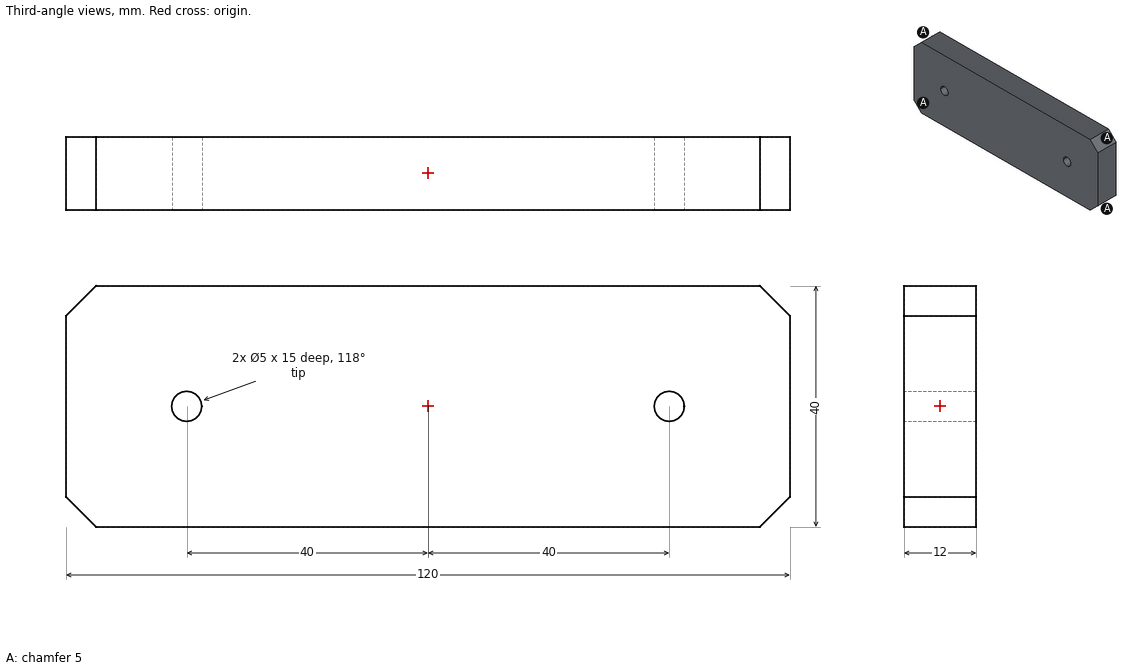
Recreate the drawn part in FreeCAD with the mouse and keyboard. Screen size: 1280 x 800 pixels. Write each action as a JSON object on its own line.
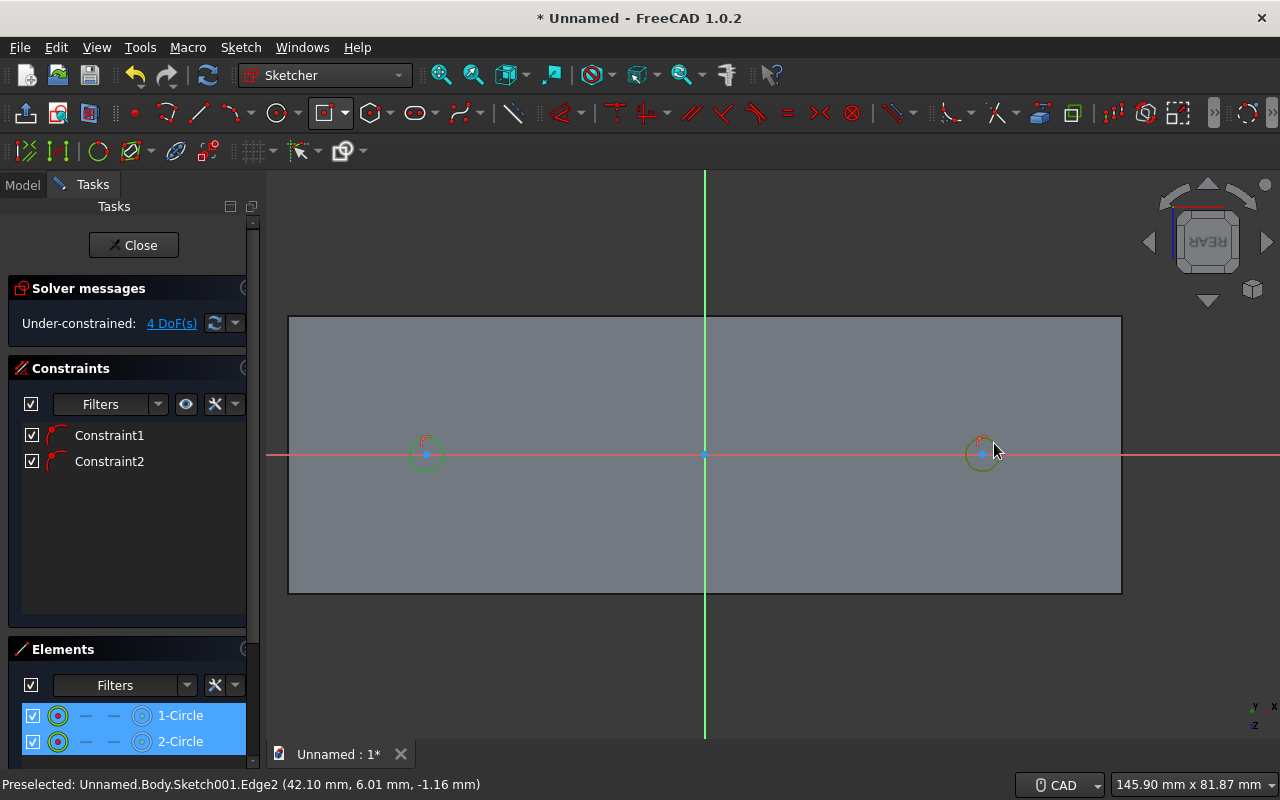
{"action": "left_click", "coordinate": [788, 114]}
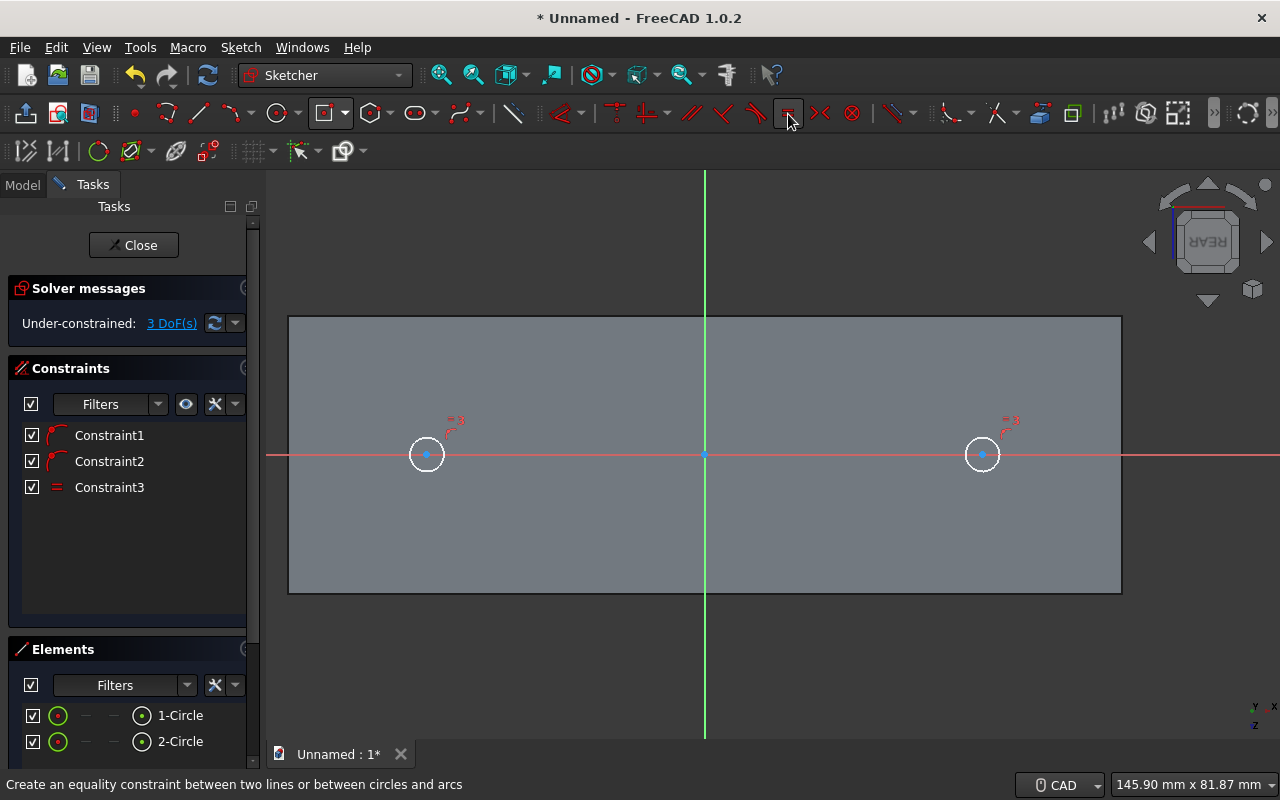
{"action": "left_click", "coordinate": [560, 114]}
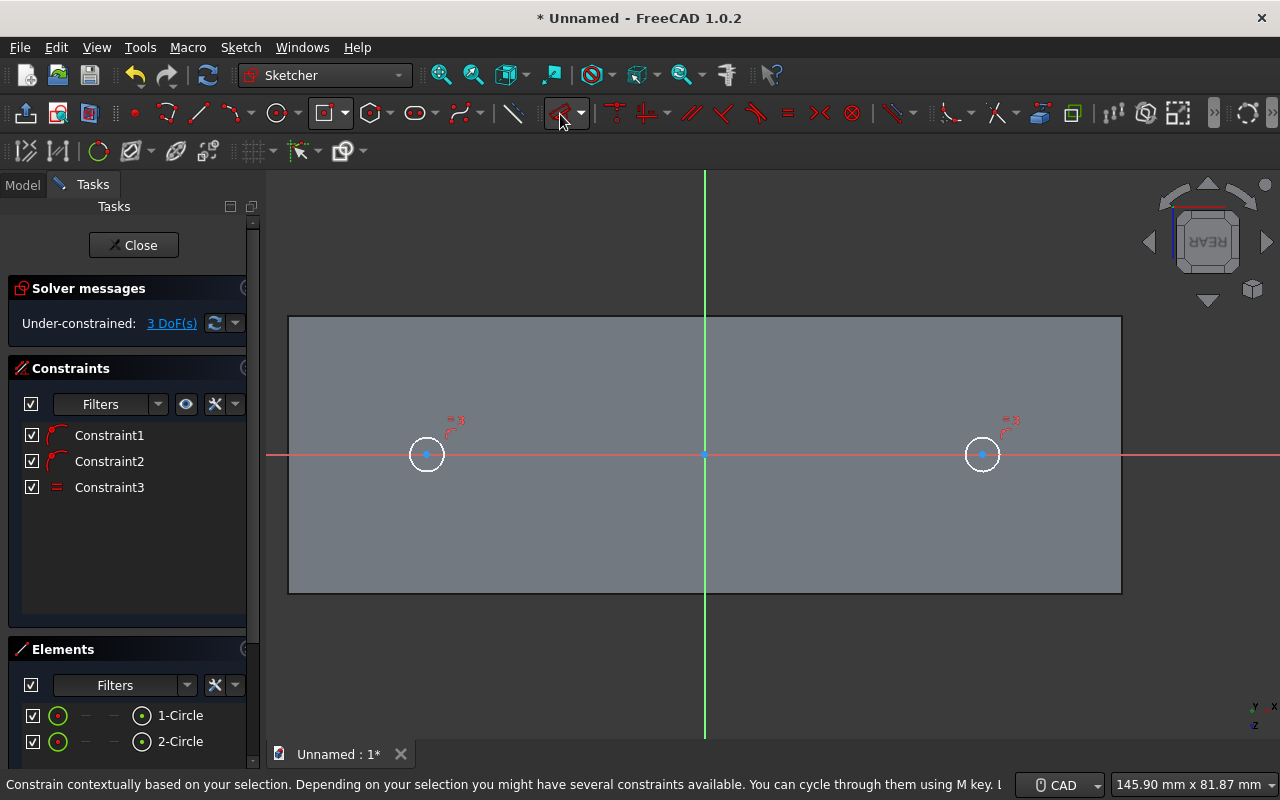
{"action": "left_click", "coordinate": [439, 443]}
{"action": "left_click", "coordinate": [462, 421]}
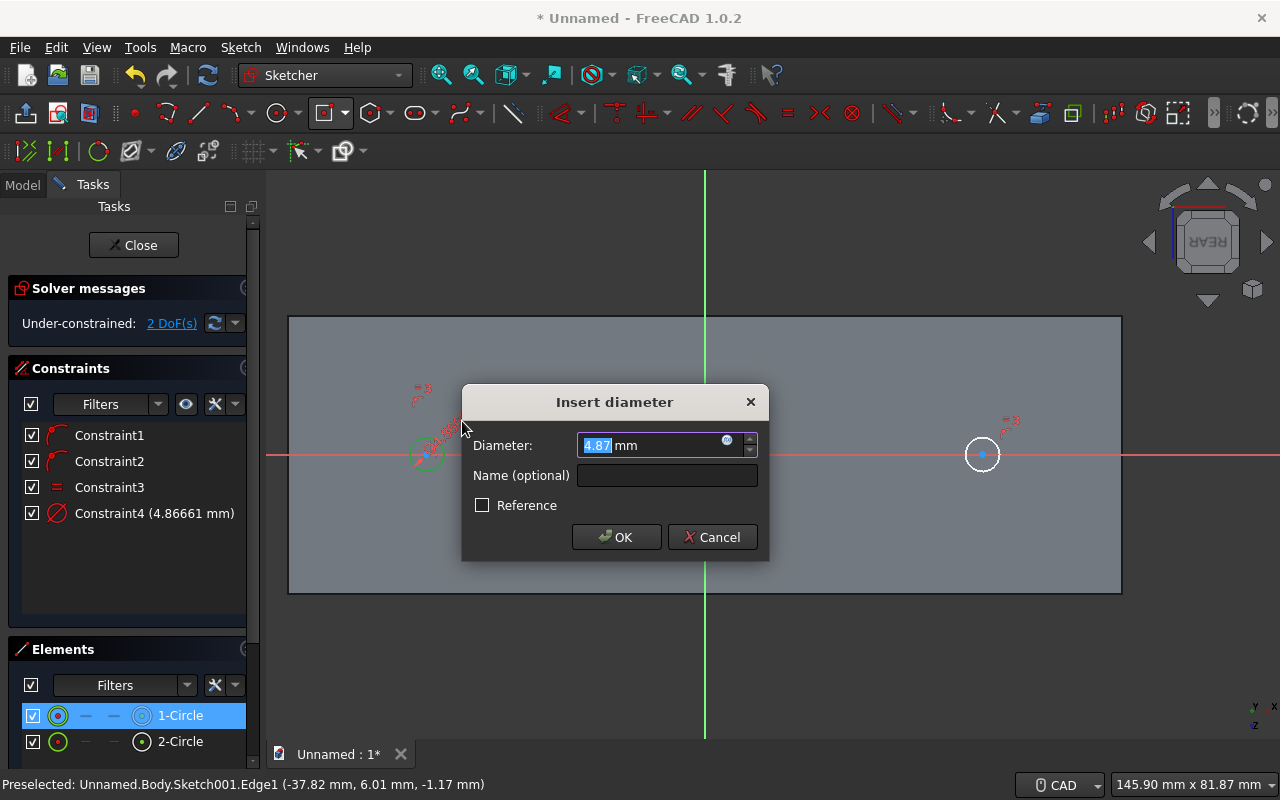
{"action": "type", "text": "5"}
{"action": "key", "text": "Return"}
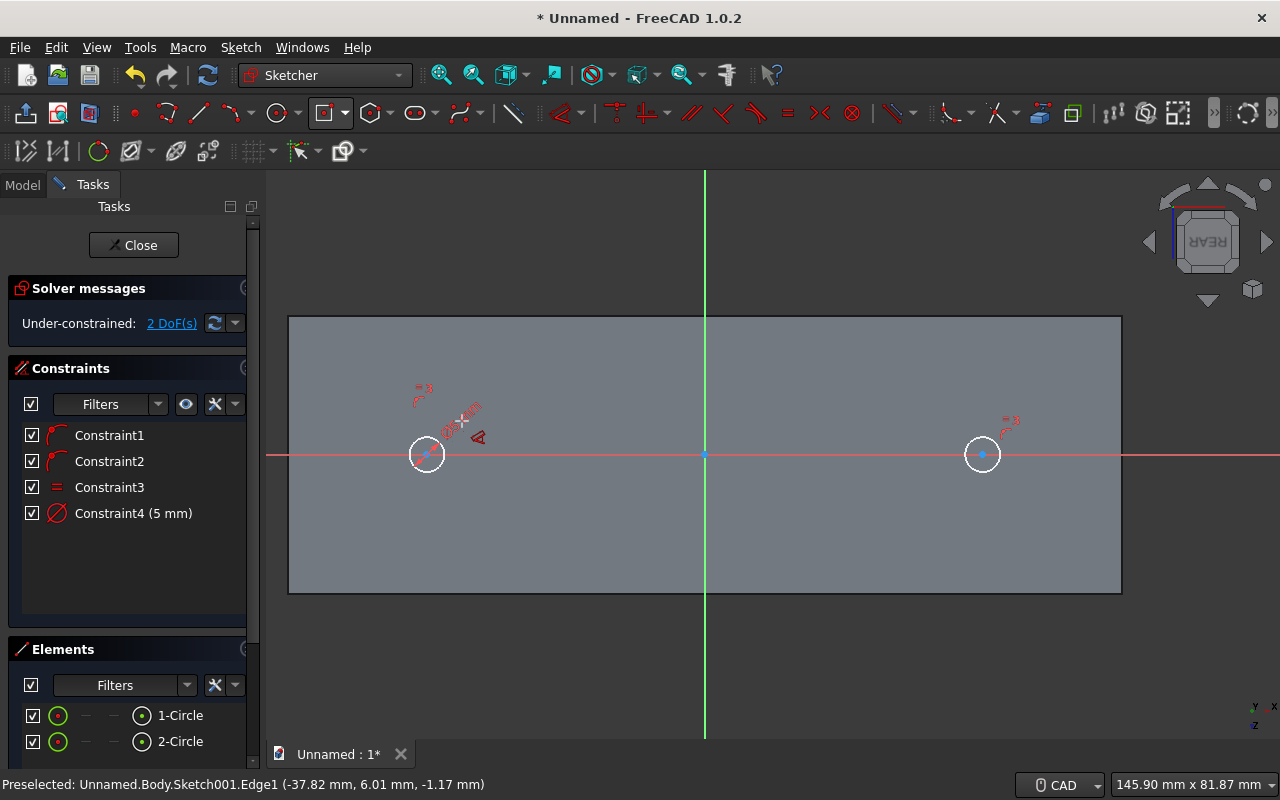
{"action": "left_click", "coordinate": [427, 455]}
{"action": "left_click", "coordinate": [566, 489]}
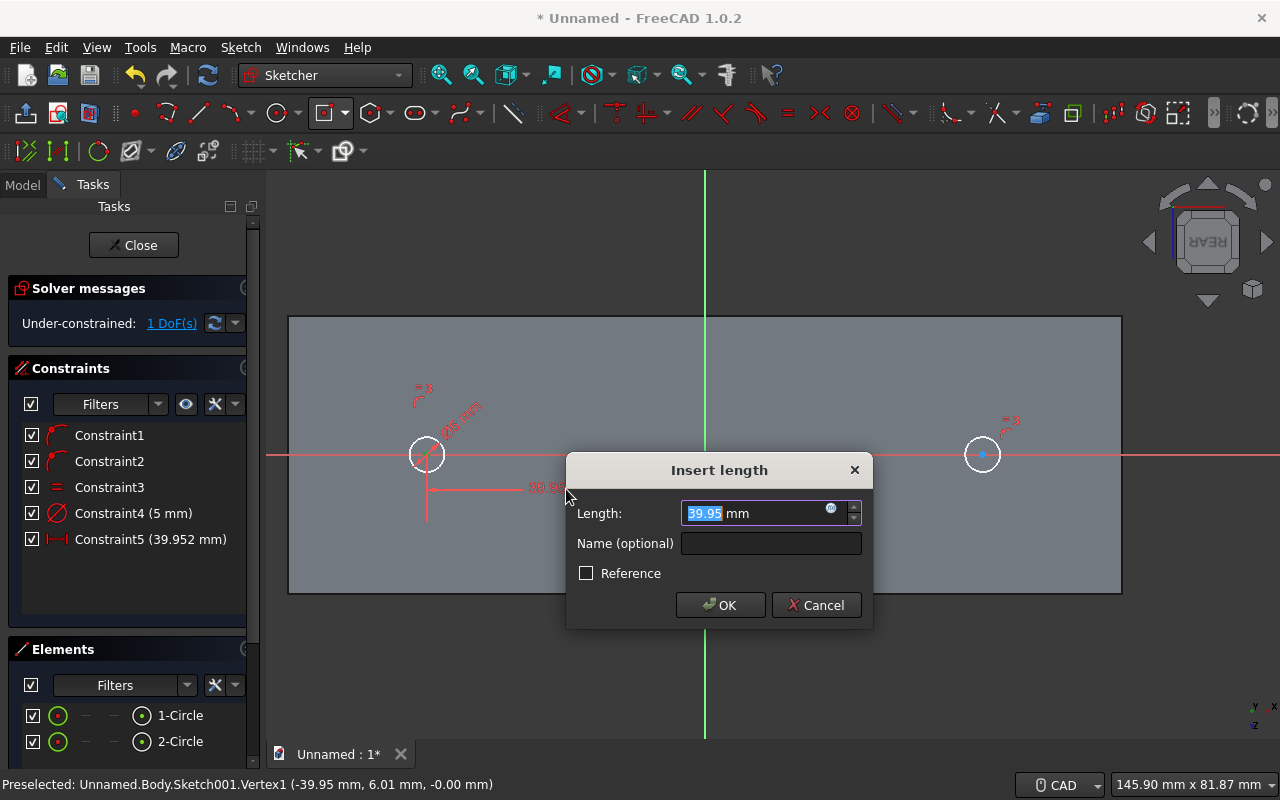
{"action": "type", "text": "40"}
{"action": "key", "text": "Return"}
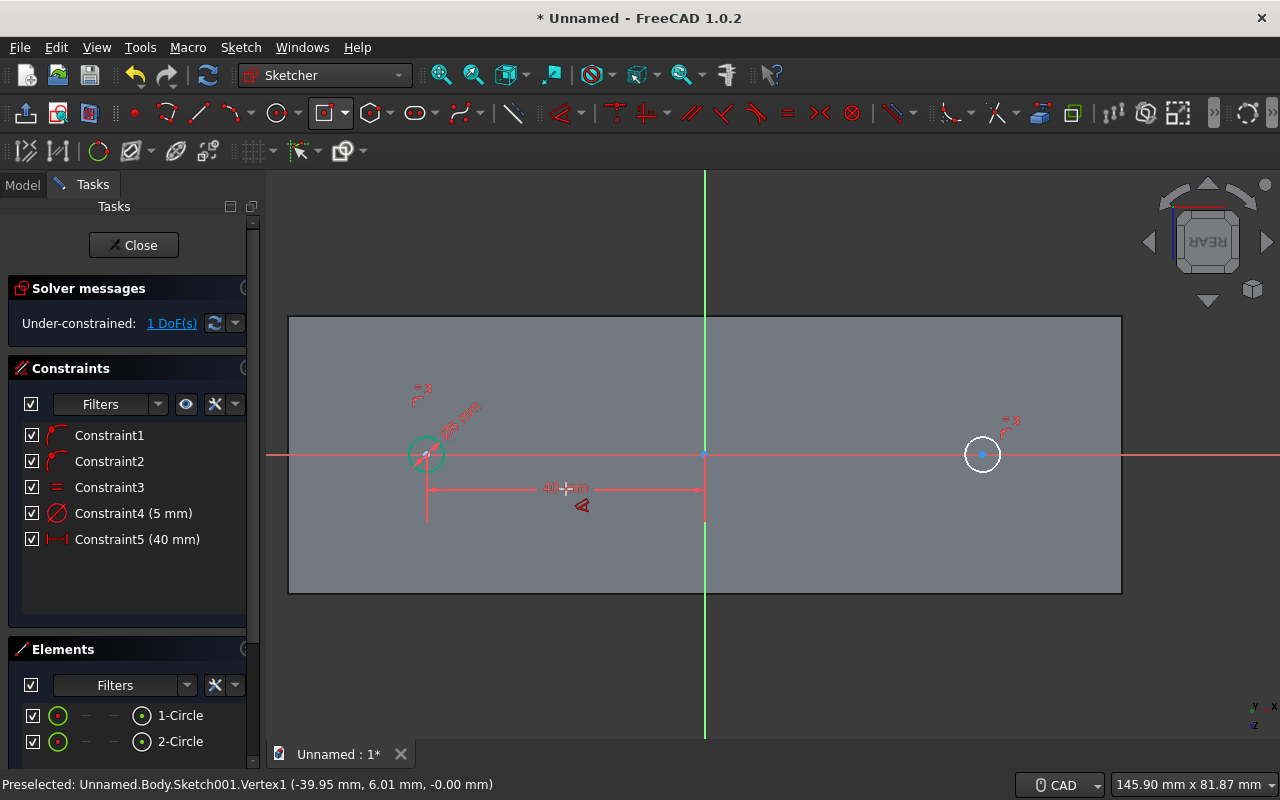
{"action": "left_click", "coordinate": [983, 455]}
{"action": "left_click", "coordinate": [844, 489]}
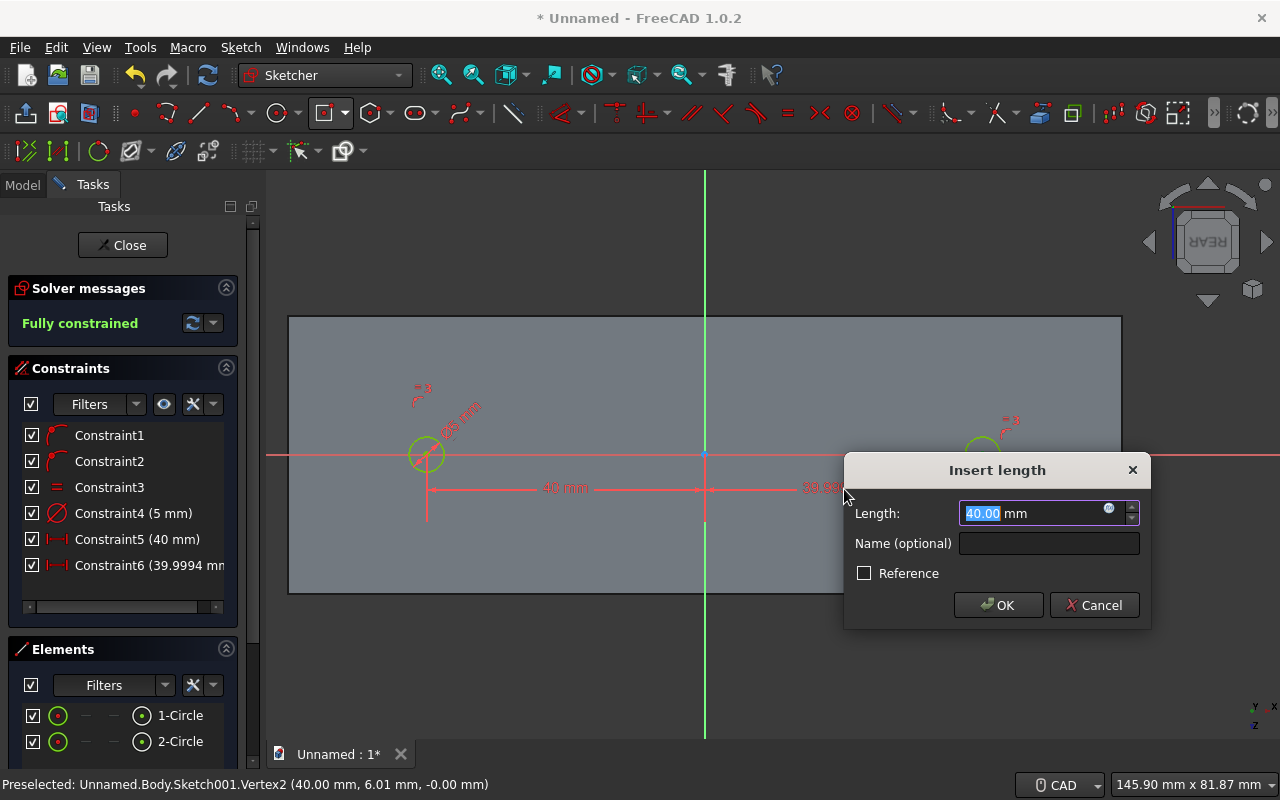
{"action": "type", "text": "40"}
{"action": "key", "text": "Return"}
{"action": "key", "text": "Escape"}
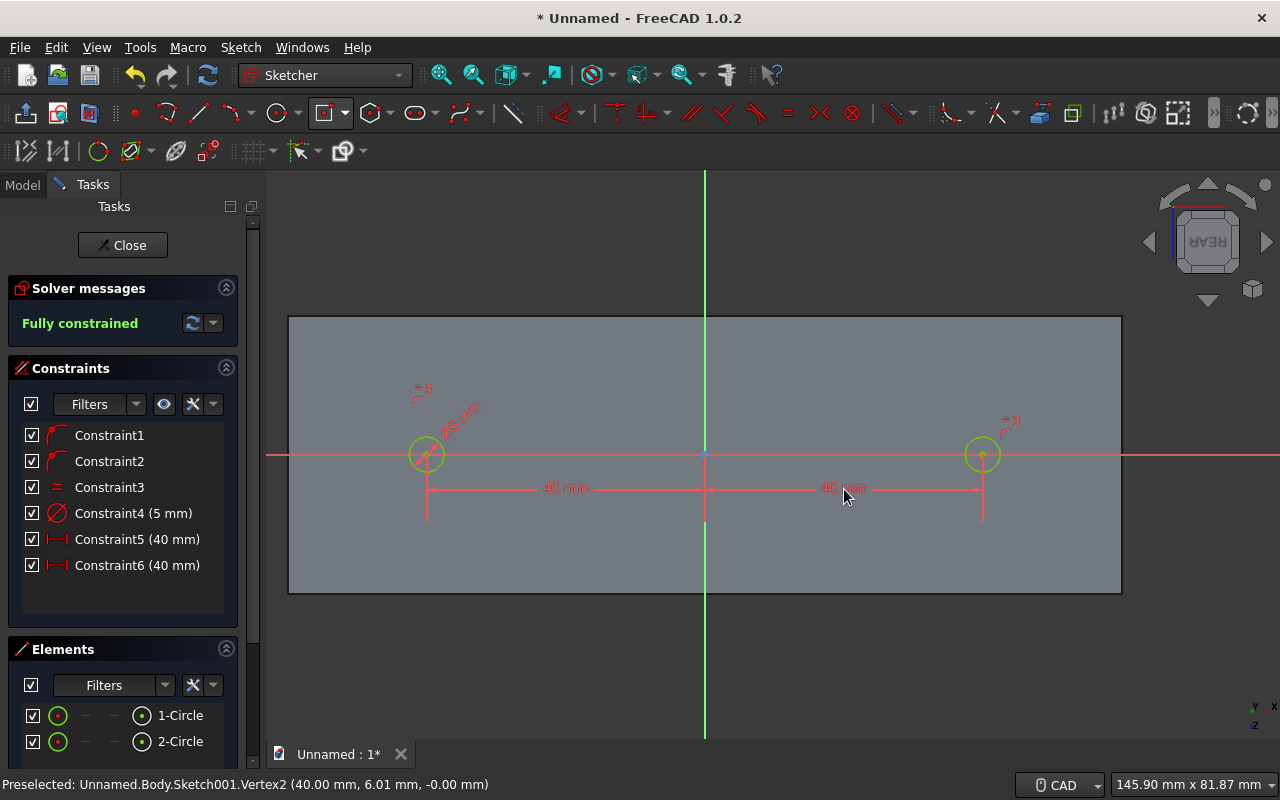
{"action": "left_click", "coordinate": [123, 245]}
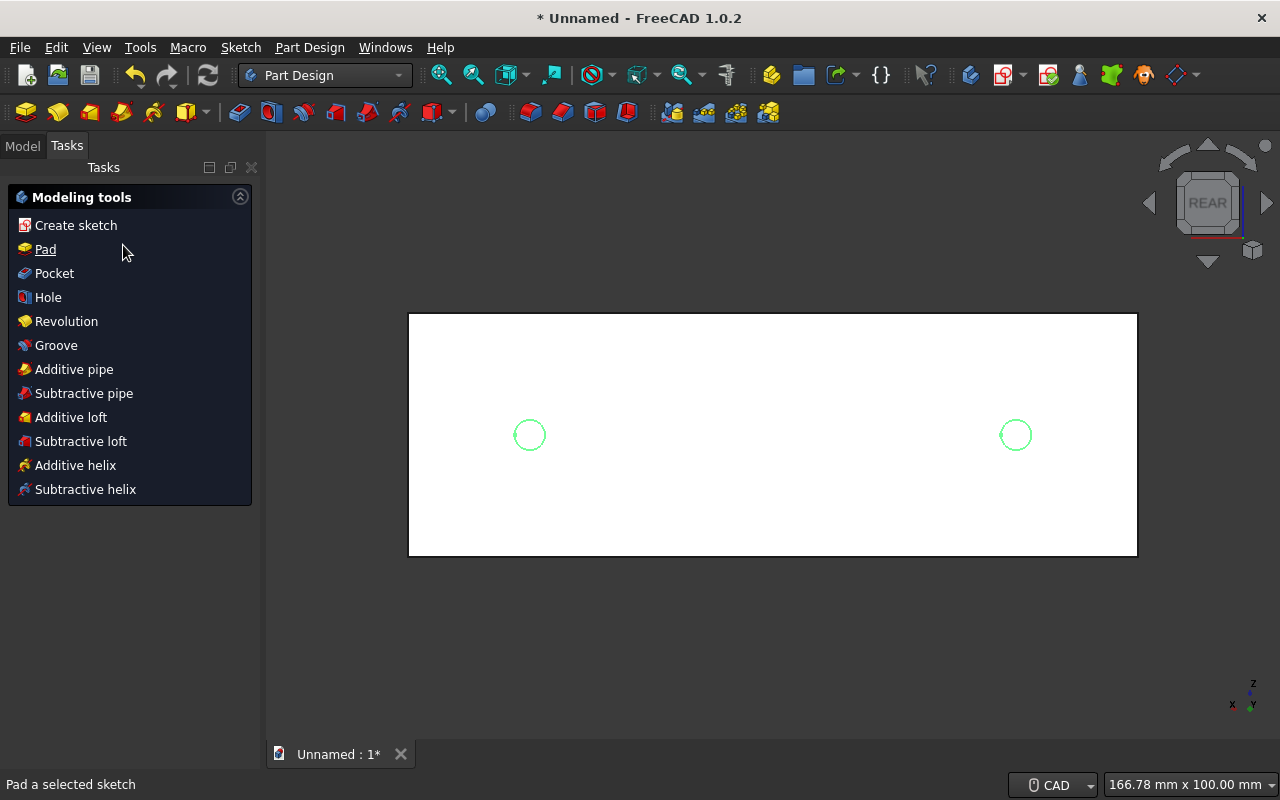
{"action": "left_click", "coordinate": [272, 112]}